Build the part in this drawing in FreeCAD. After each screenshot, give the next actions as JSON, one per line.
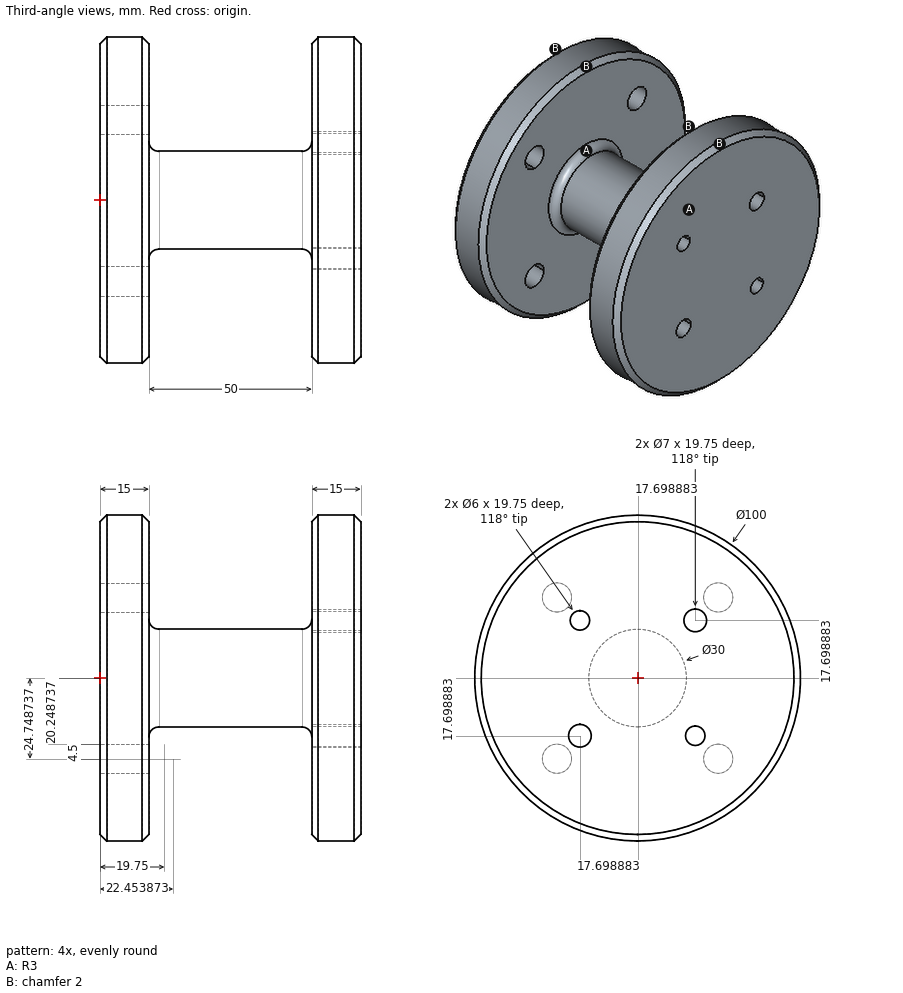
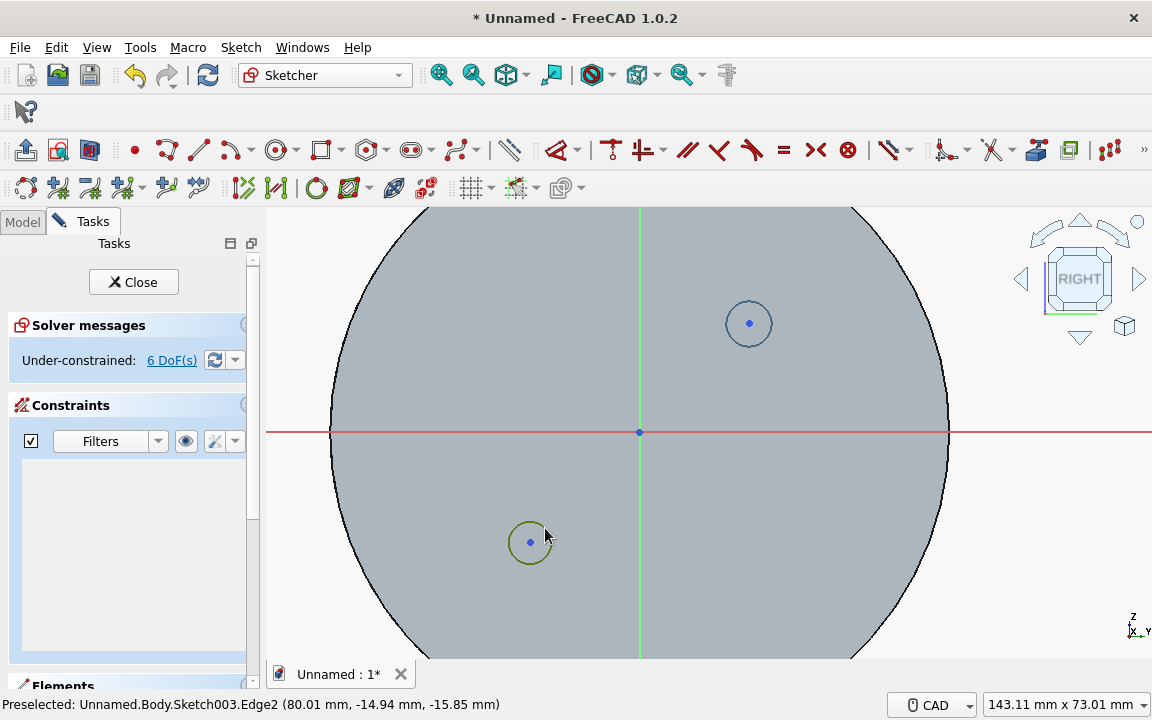
{"action": "left_click", "coordinate": [784, 150]}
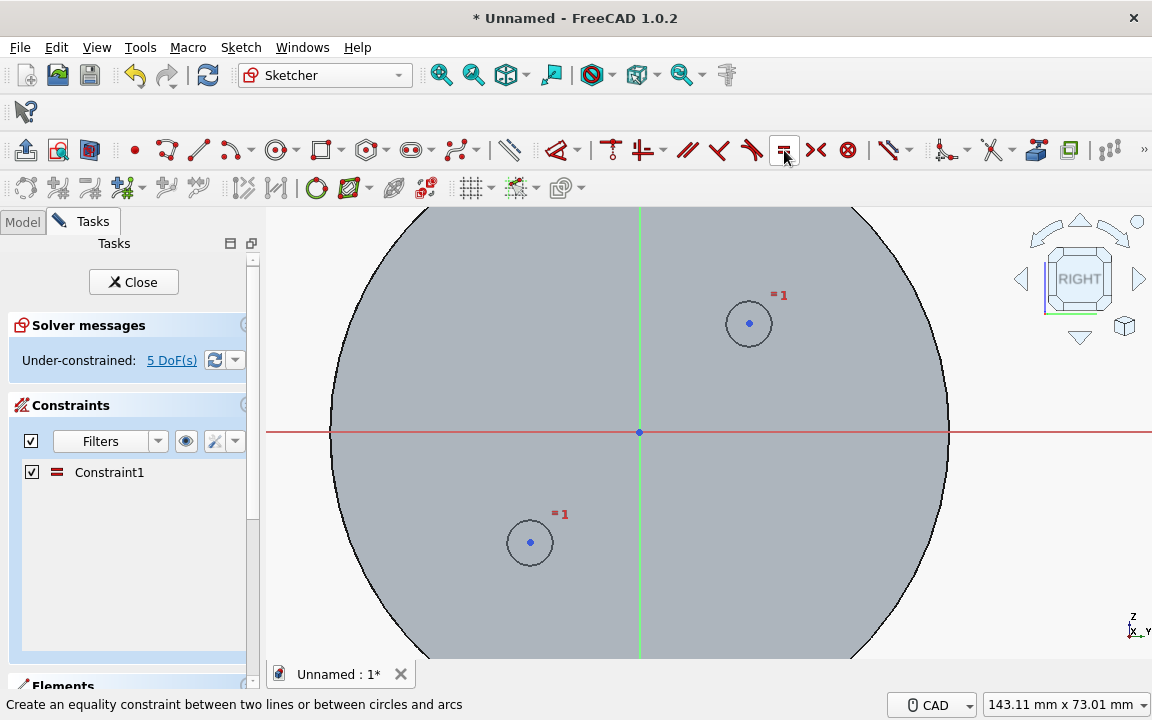
{"action": "left_click", "coordinate": [556, 150]}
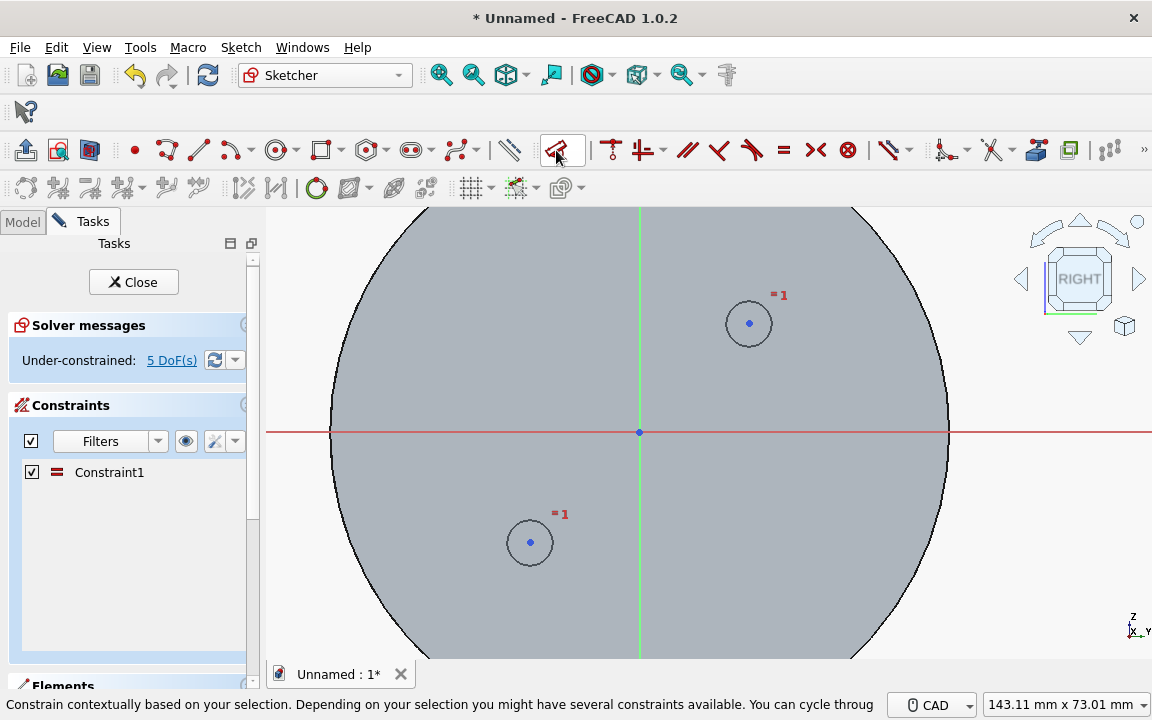
{"action": "left_click", "coordinate": [765, 308]}
{"action": "left_click", "coordinate": [788, 285]}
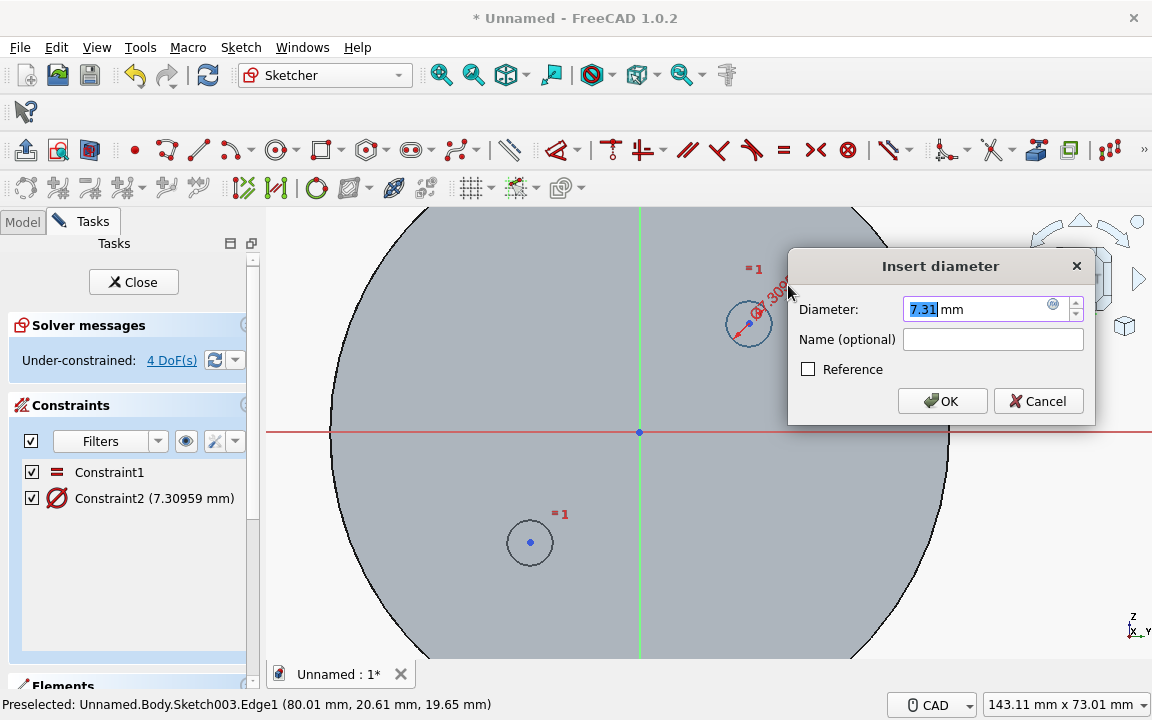
{"action": "type", "text": "7"}
{"action": "key", "text": "Return"}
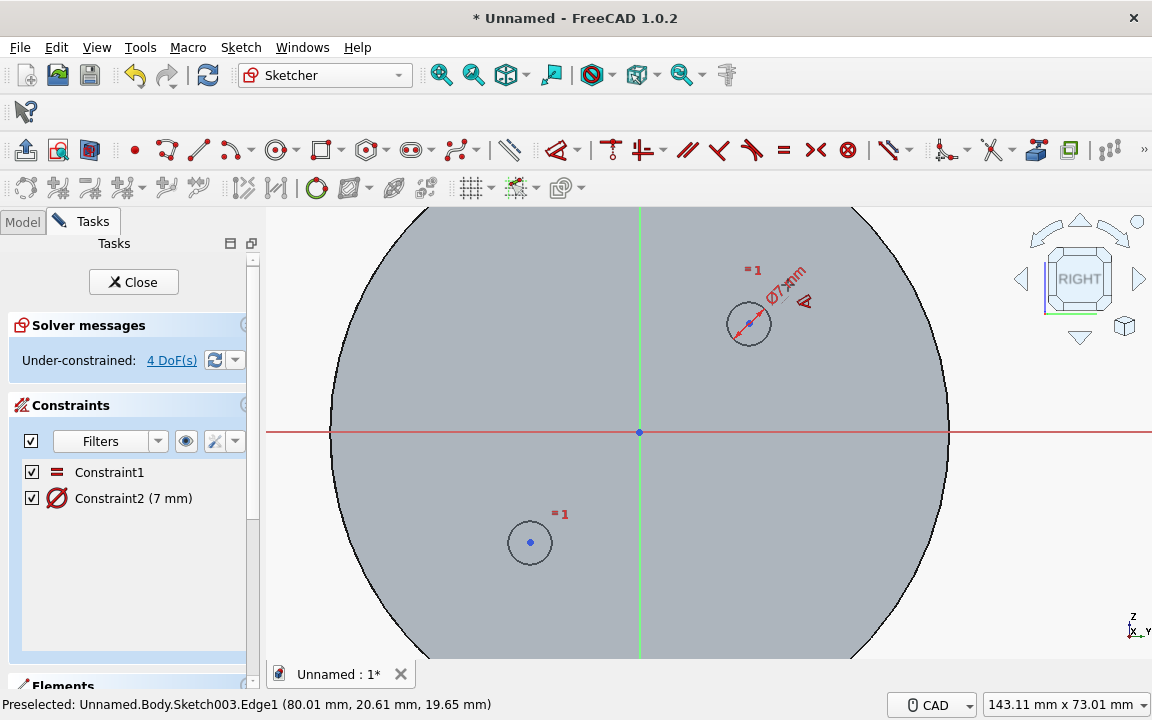
{"action": "left_click", "coordinate": [749, 324]}
{"action": "left_click", "coordinate": [694, 290]}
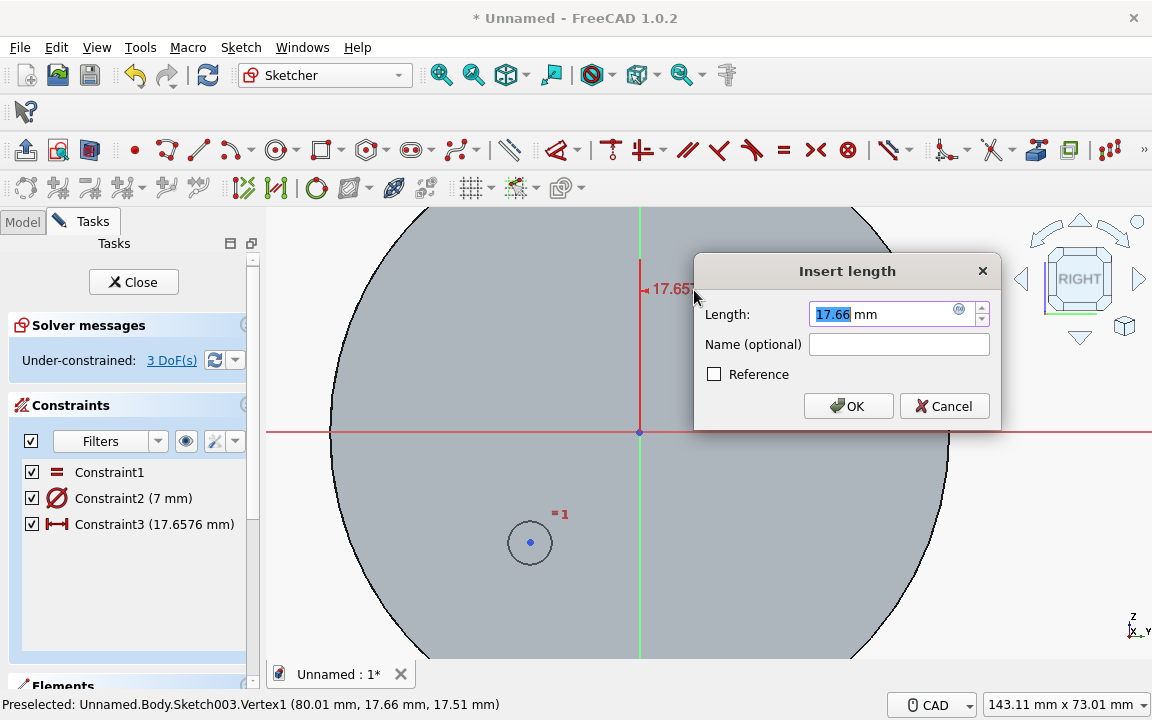
{"action": "type", "text": "17.698883"}
{"action": "key", "text": "Return"}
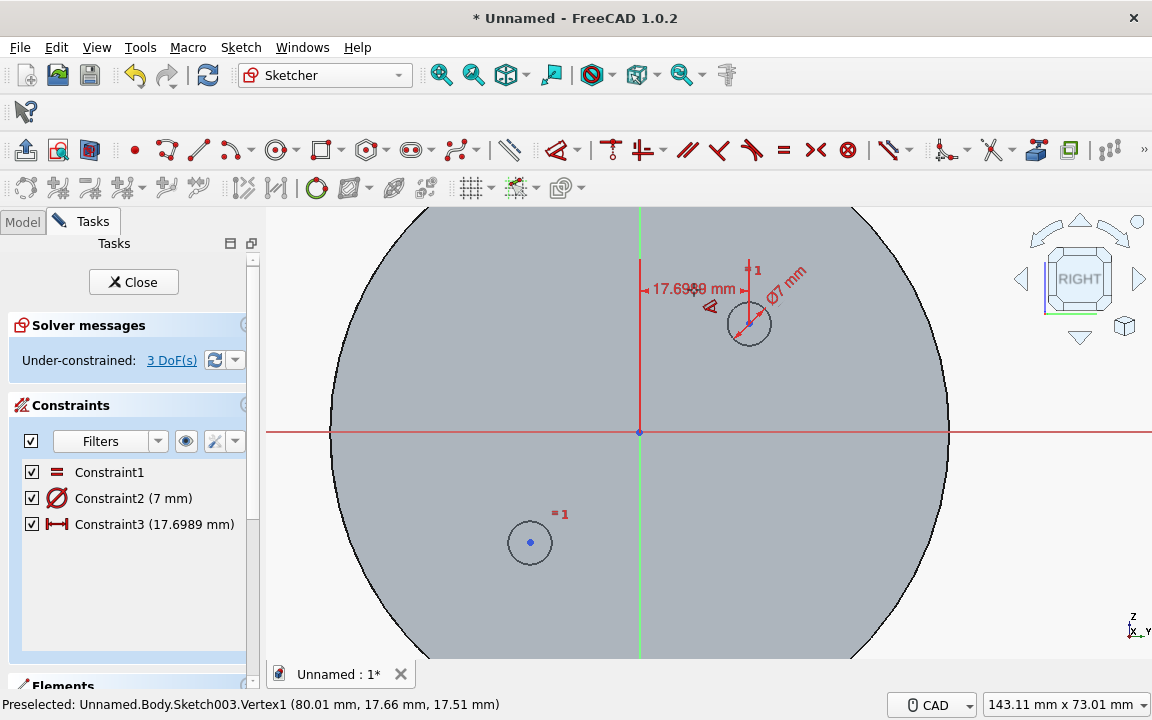
{"action": "left_click", "coordinate": [749, 324]}
{"action": "left_click", "coordinate": [783, 378]}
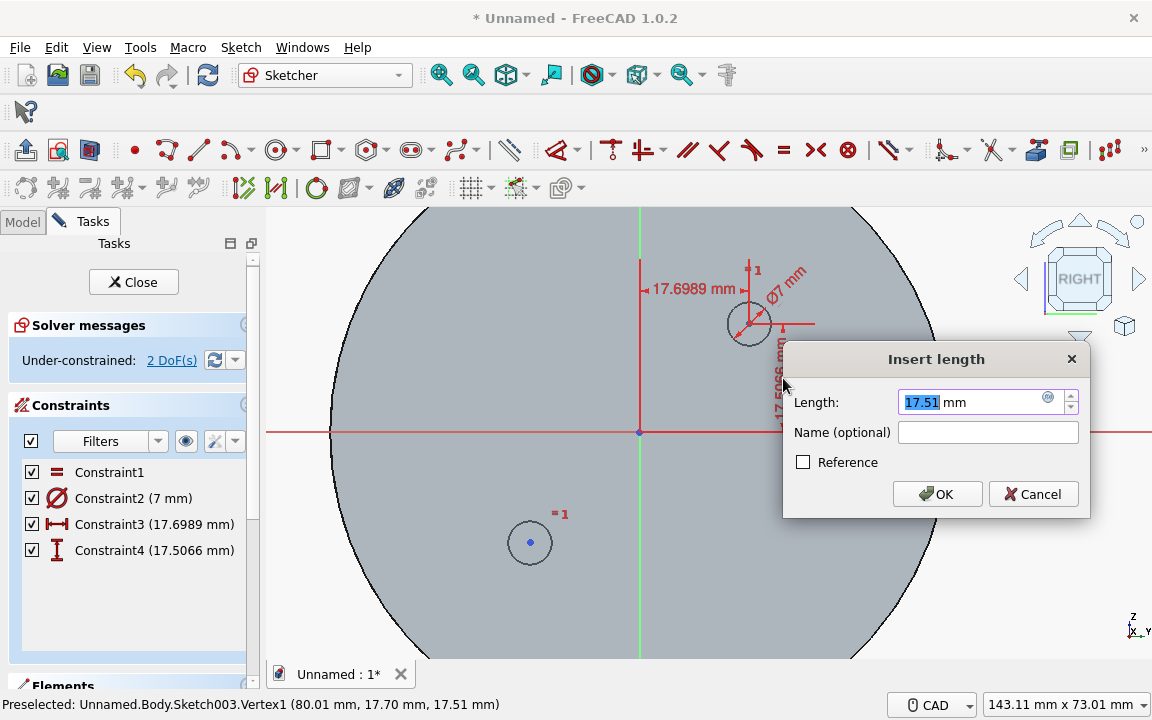
{"action": "type", "text": "17.698883"}
{"action": "key", "text": "Return"}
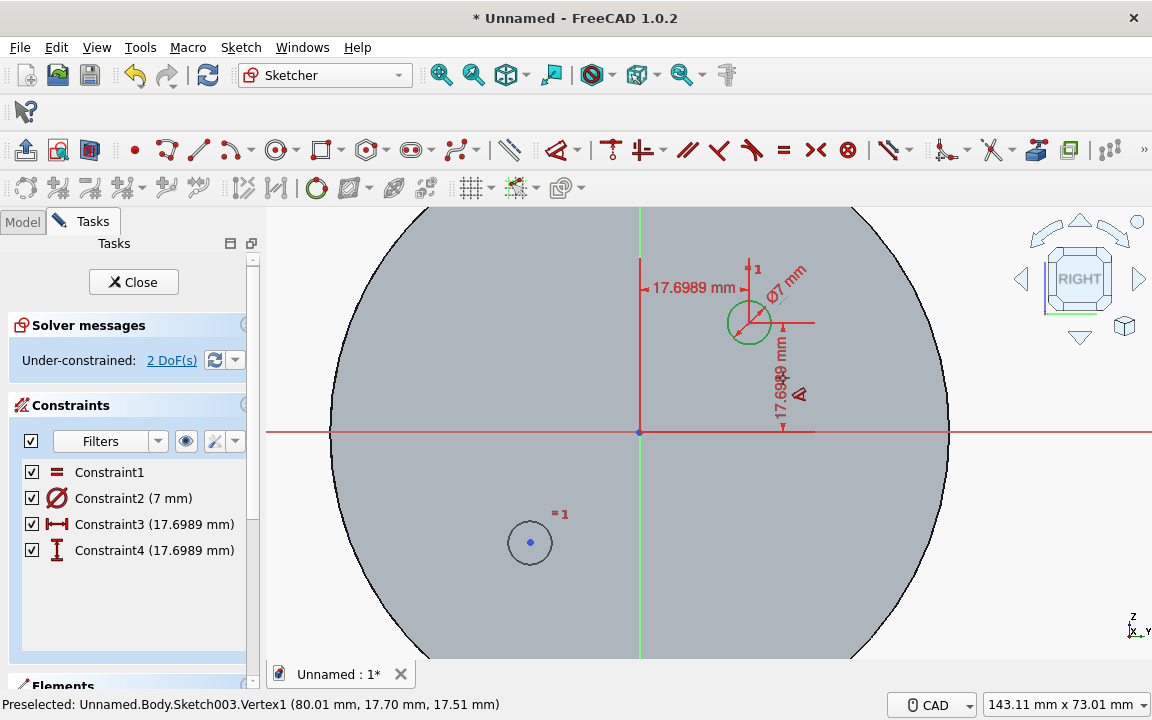
{"action": "left_click", "coordinate": [530, 543]}
{"action": "left_click", "coordinate": [585, 577]}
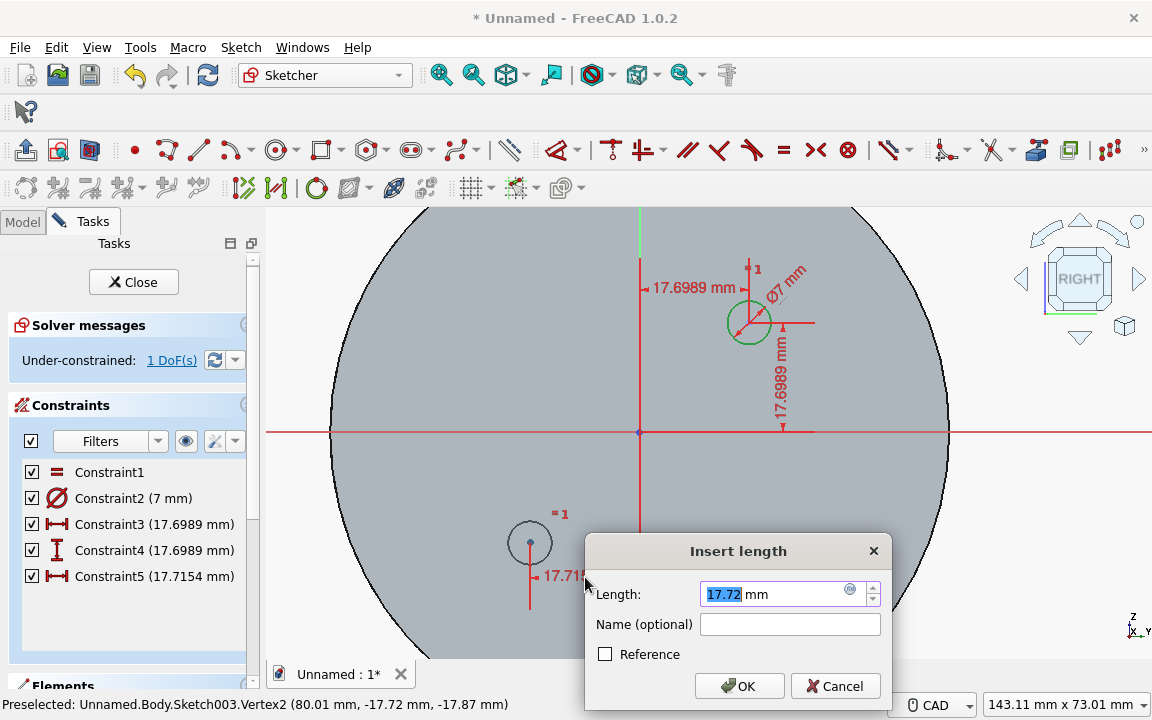
{"action": "type", "text": "17.698883"}
{"action": "key", "text": "Return"}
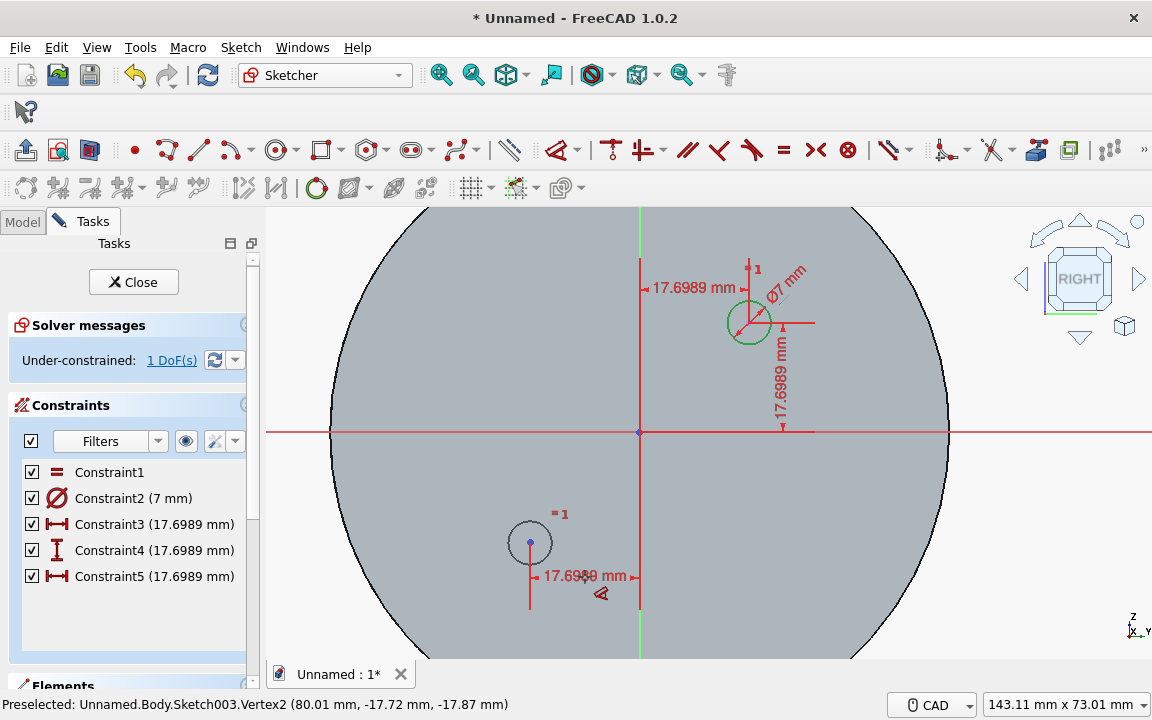
{"action": "left_click", "coordinate": [530, 543]}
{"action": "left_click", "coordinate": [496, 488]}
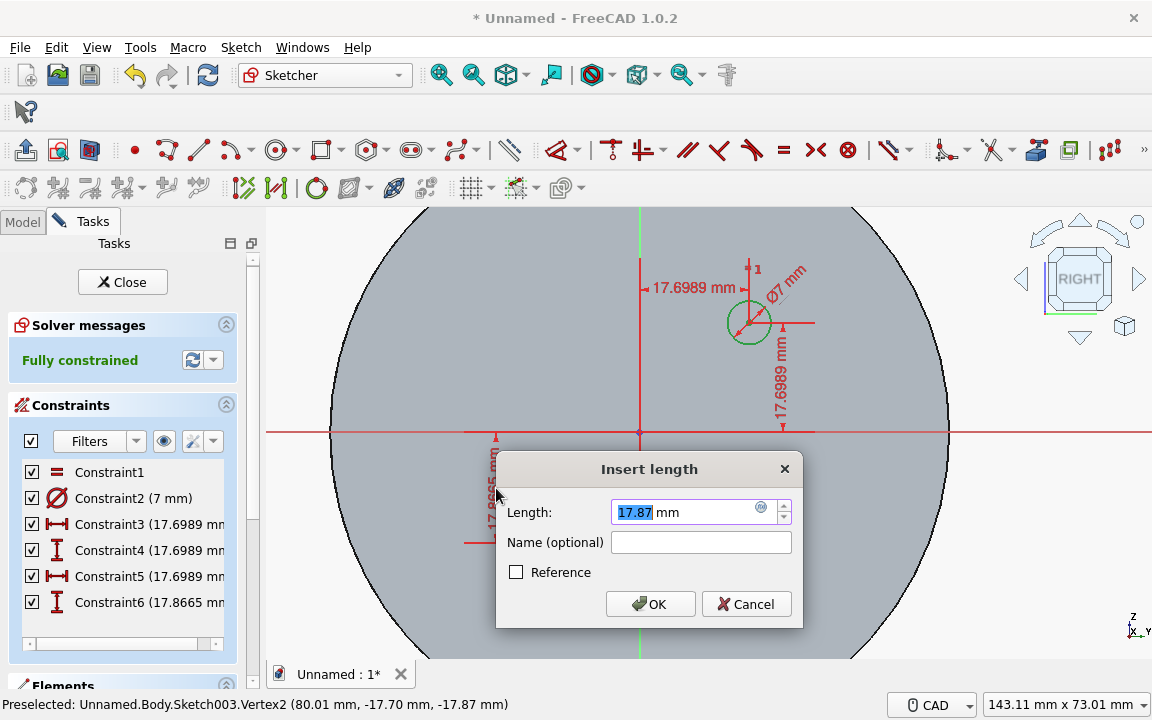
{"action": "type", "text": "17.698883"}
{"action": "key", "text": "Return"}
{"action": "key", "text": "Escape"}